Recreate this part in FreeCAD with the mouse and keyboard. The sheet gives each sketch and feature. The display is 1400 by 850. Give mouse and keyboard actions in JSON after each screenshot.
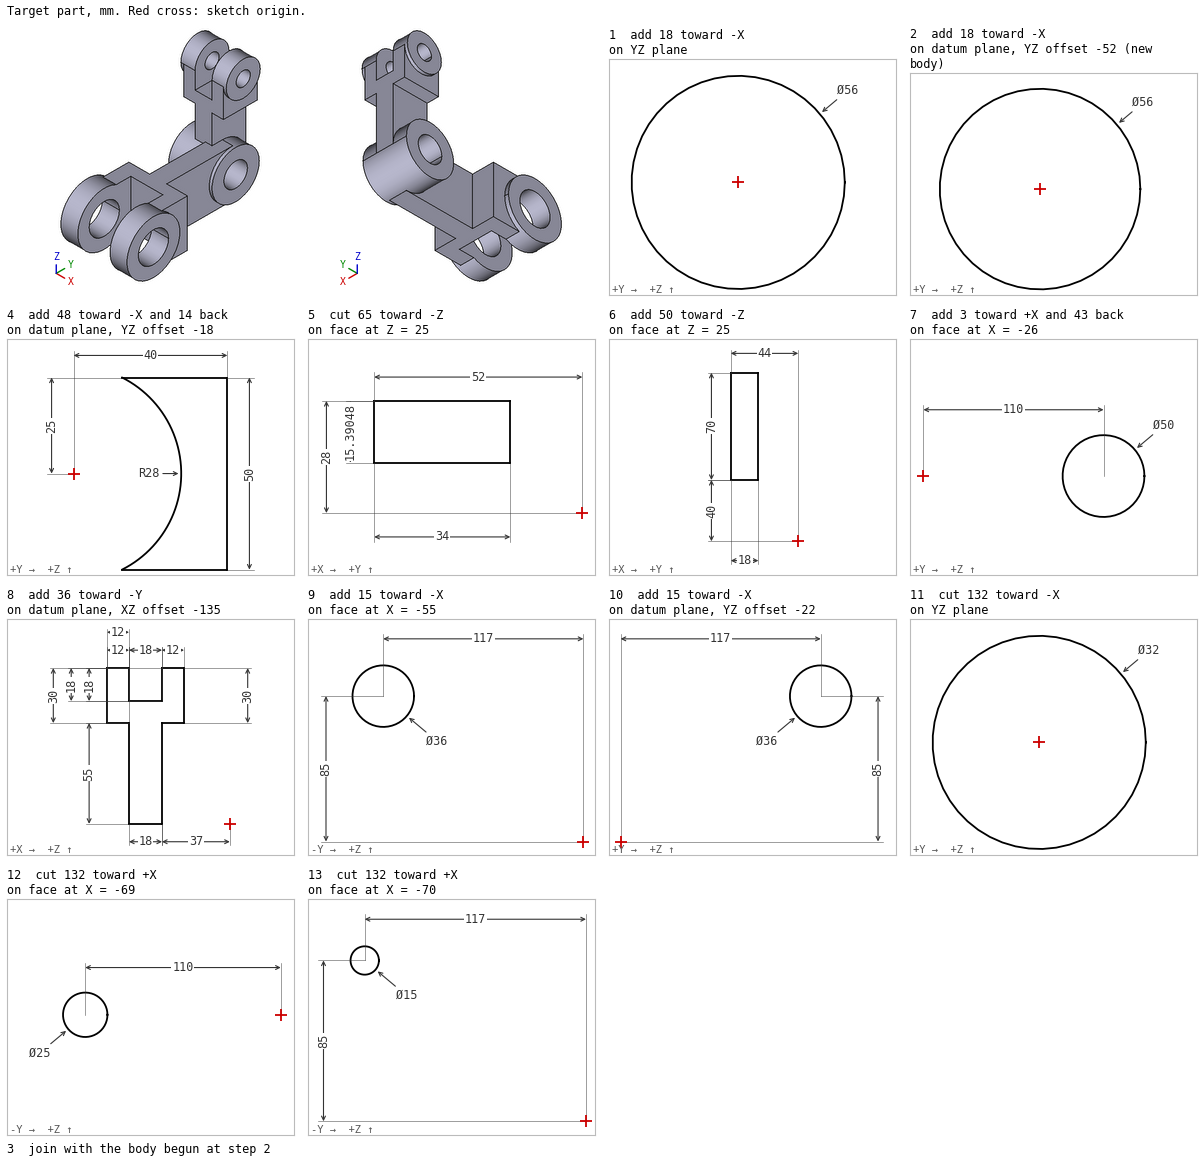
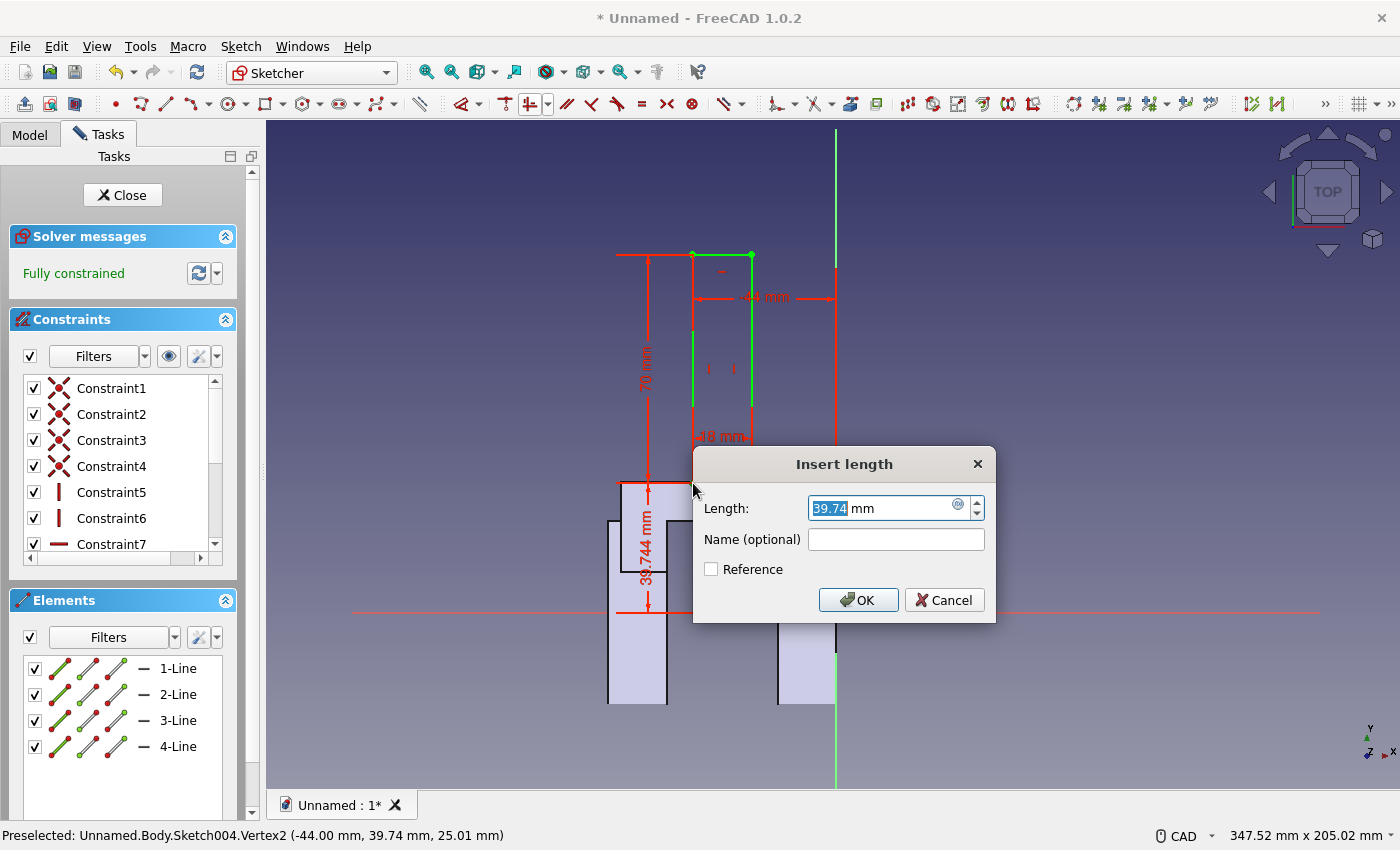
{"action": "type", "text": "40"}
{"action": "key", "text": "Return"}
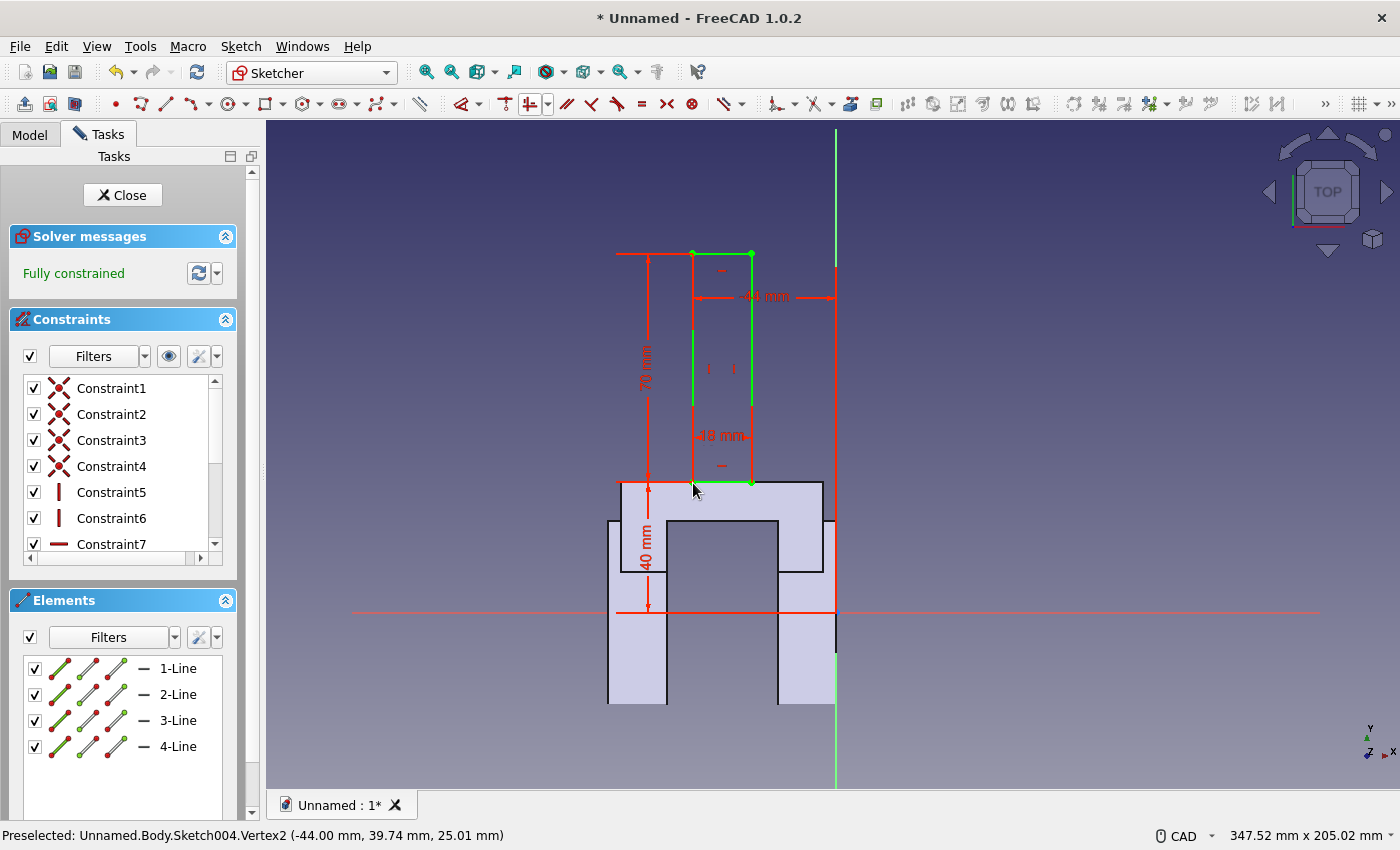
{"action": "left_click", "coordinate": [123, 195]}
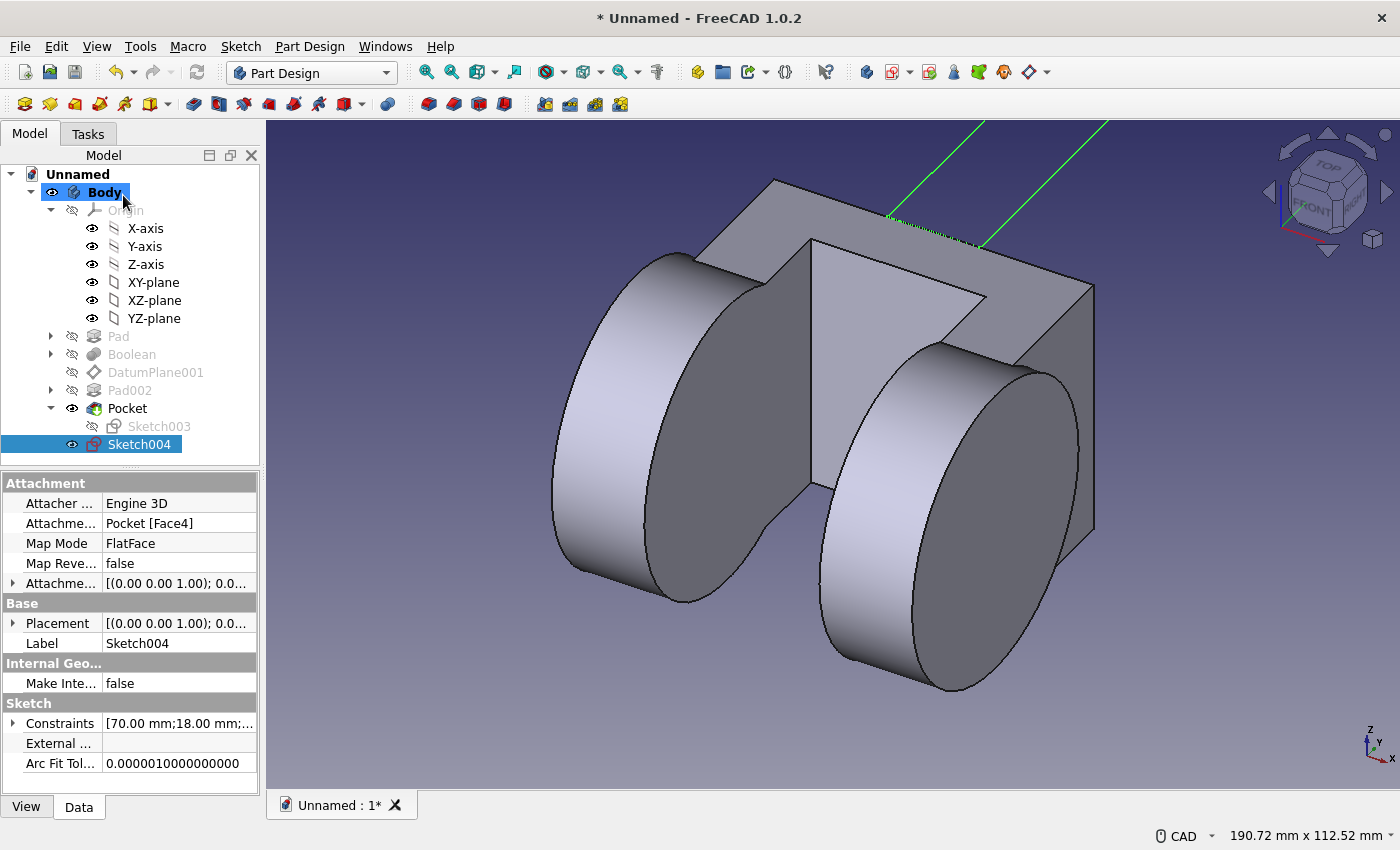
{"action": "left_click", "coordinate": [25, 104]}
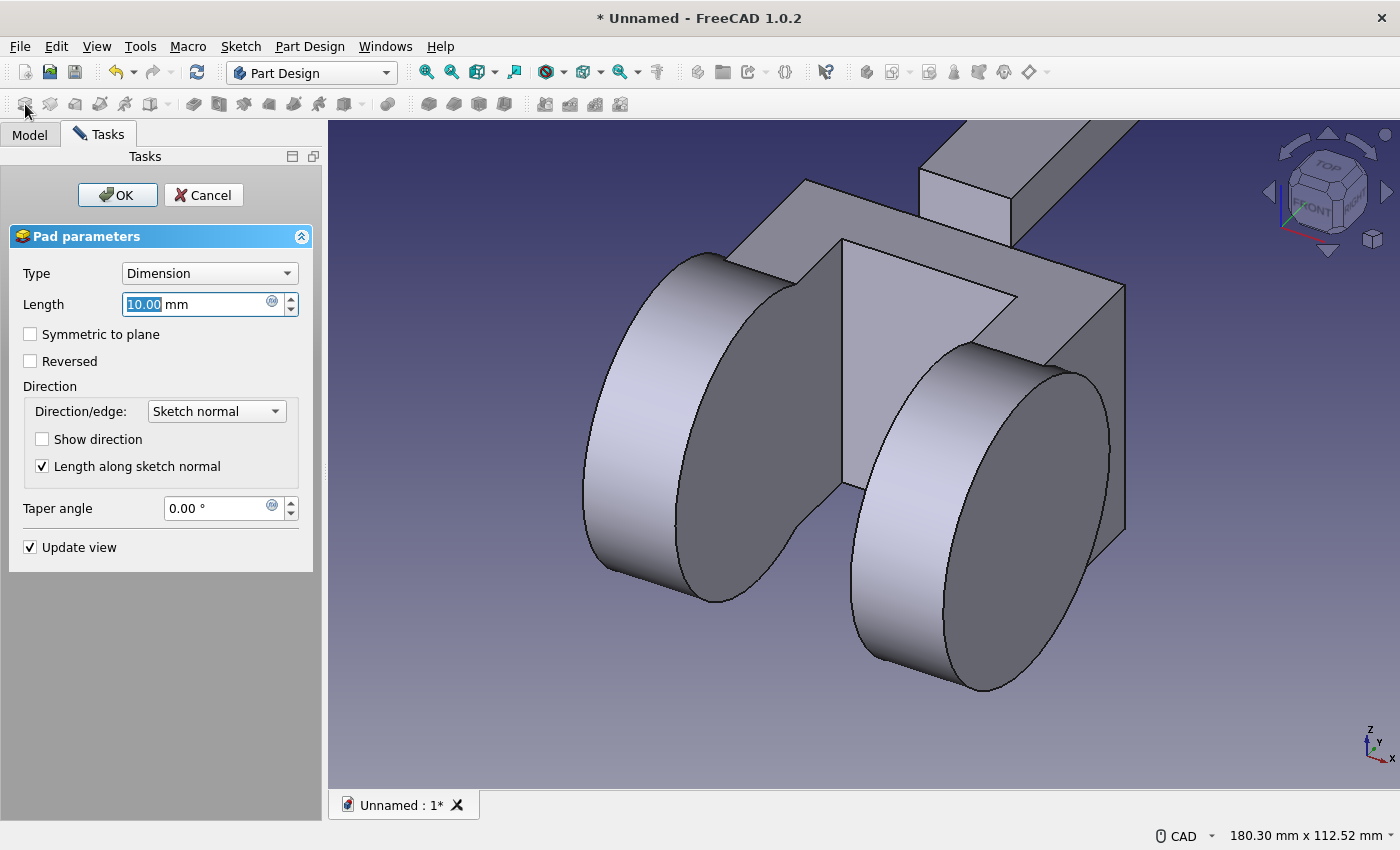
{"action": "type", "text": "50"}
{"action": "key", "text": "Tab"}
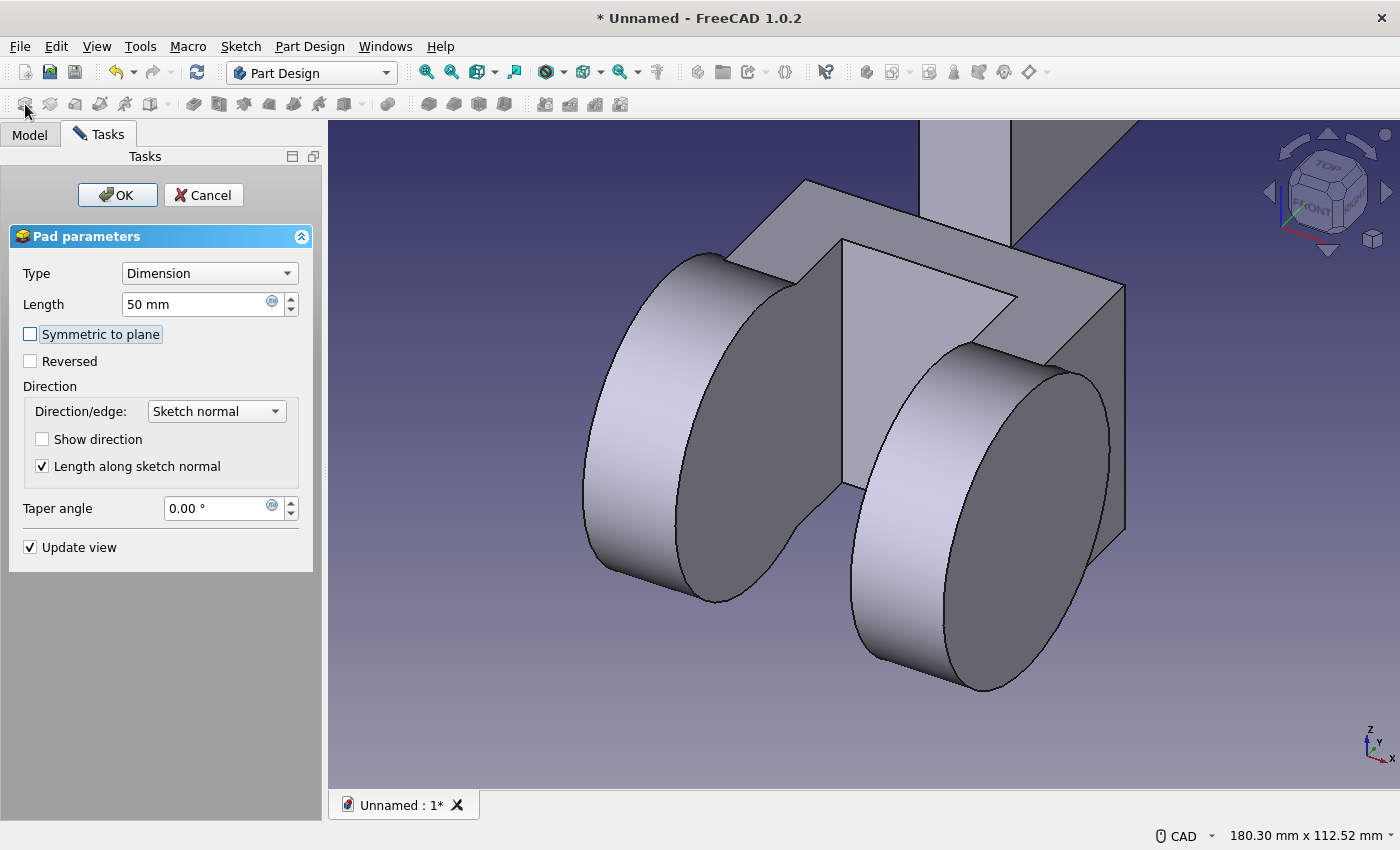
{"action": "left_click", "coordinate": [31, 361]}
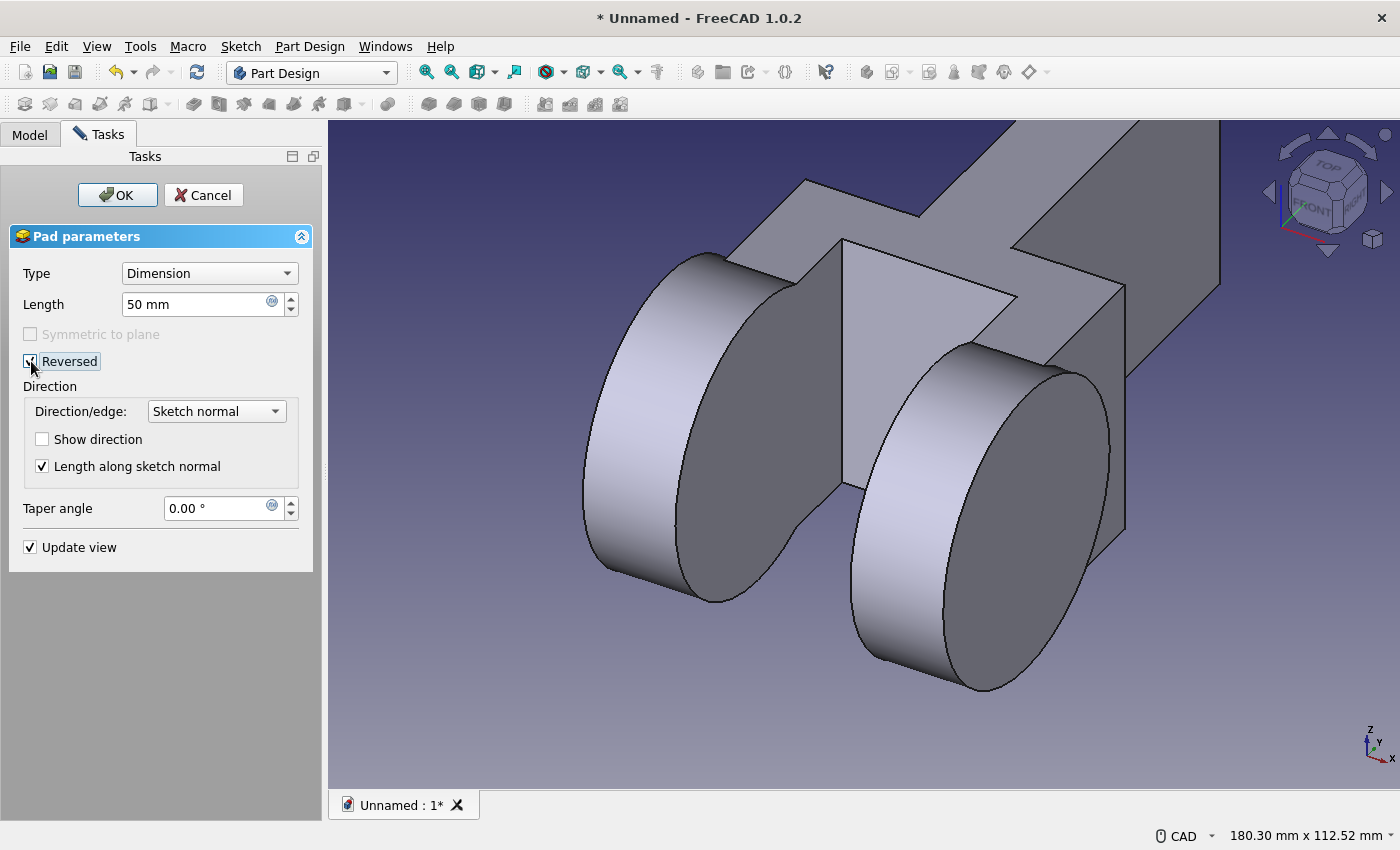
{"action": "left_click", "coordinate": [118, 195]}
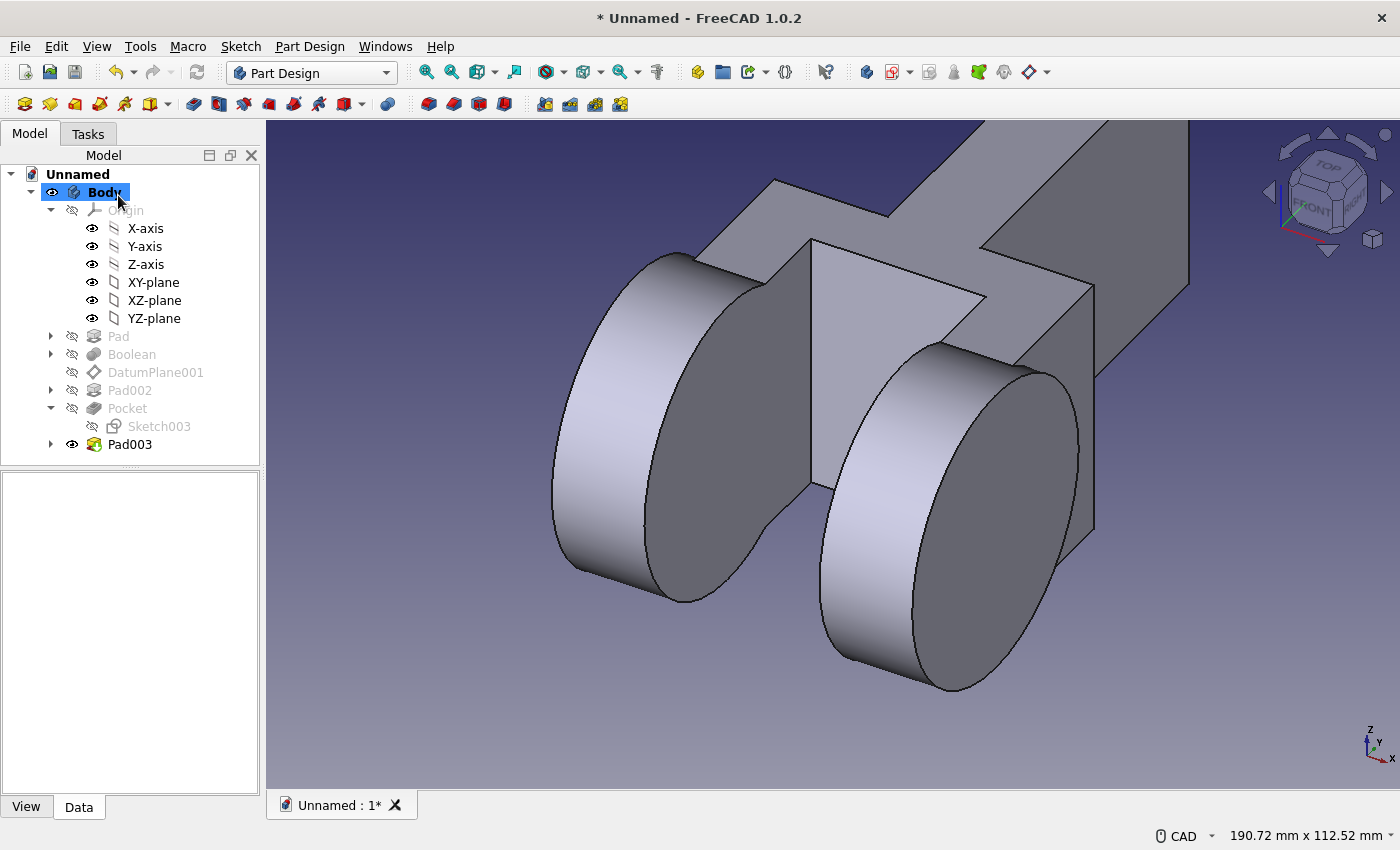
{"action": "key", "text": "v f"}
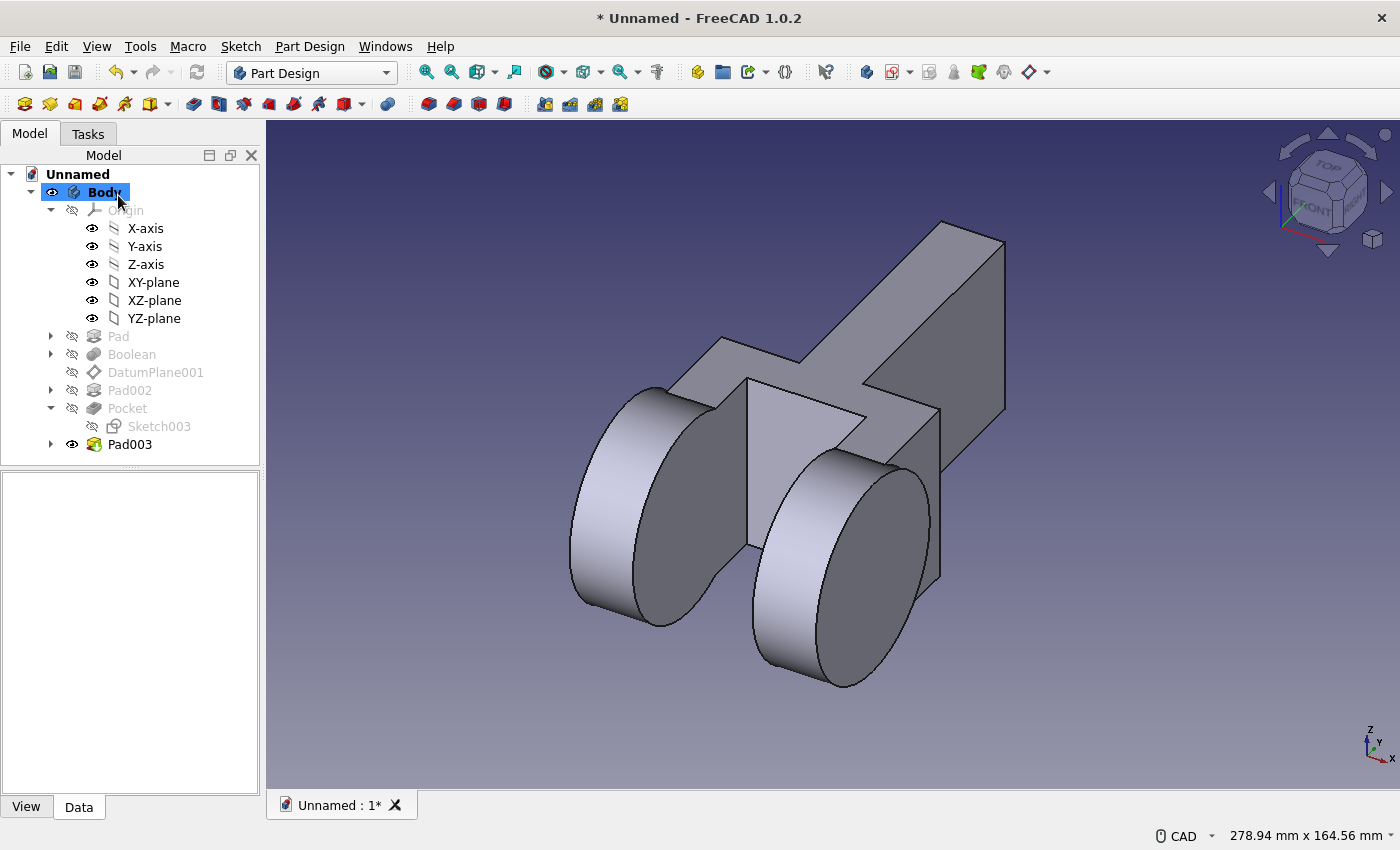
{"action": "left_click", "coordinate": [954, 375]}